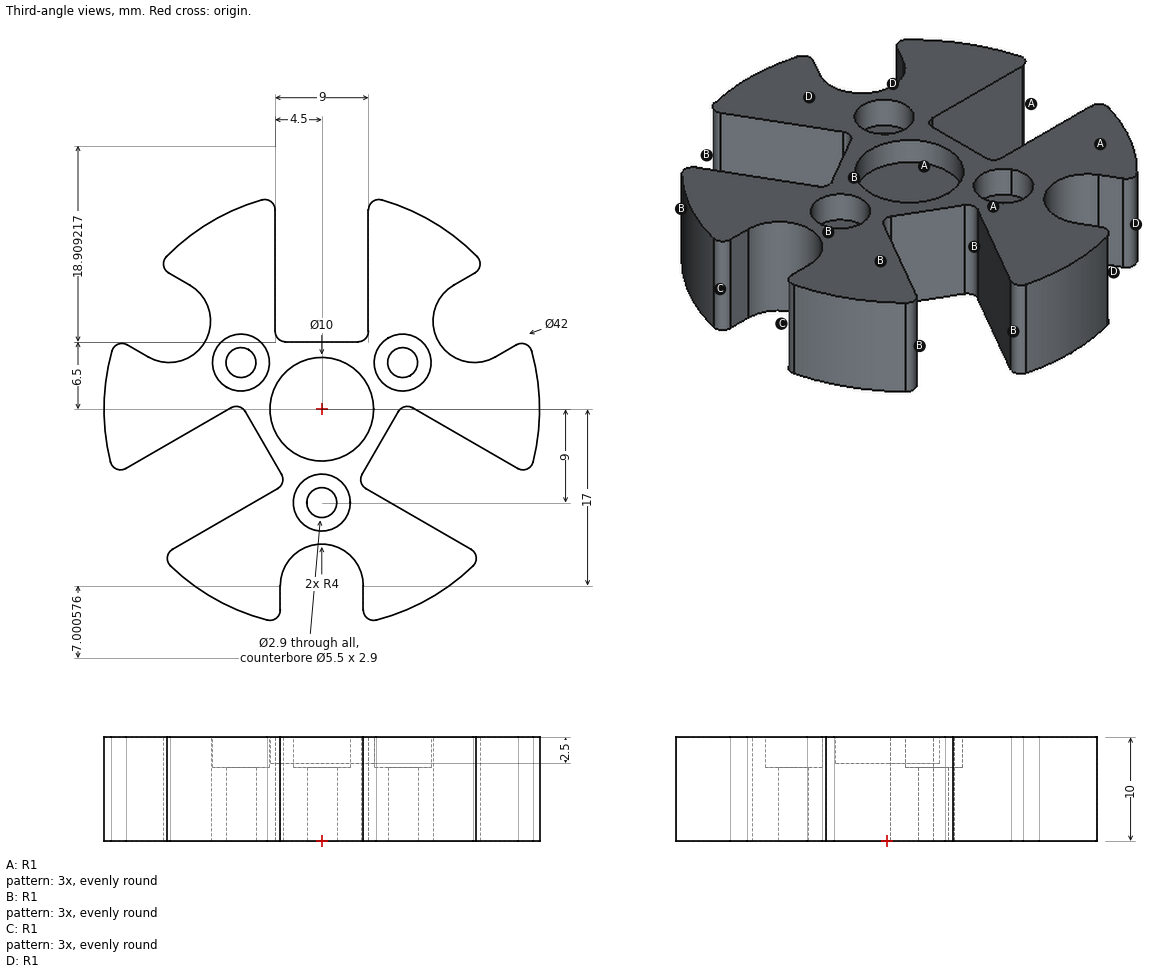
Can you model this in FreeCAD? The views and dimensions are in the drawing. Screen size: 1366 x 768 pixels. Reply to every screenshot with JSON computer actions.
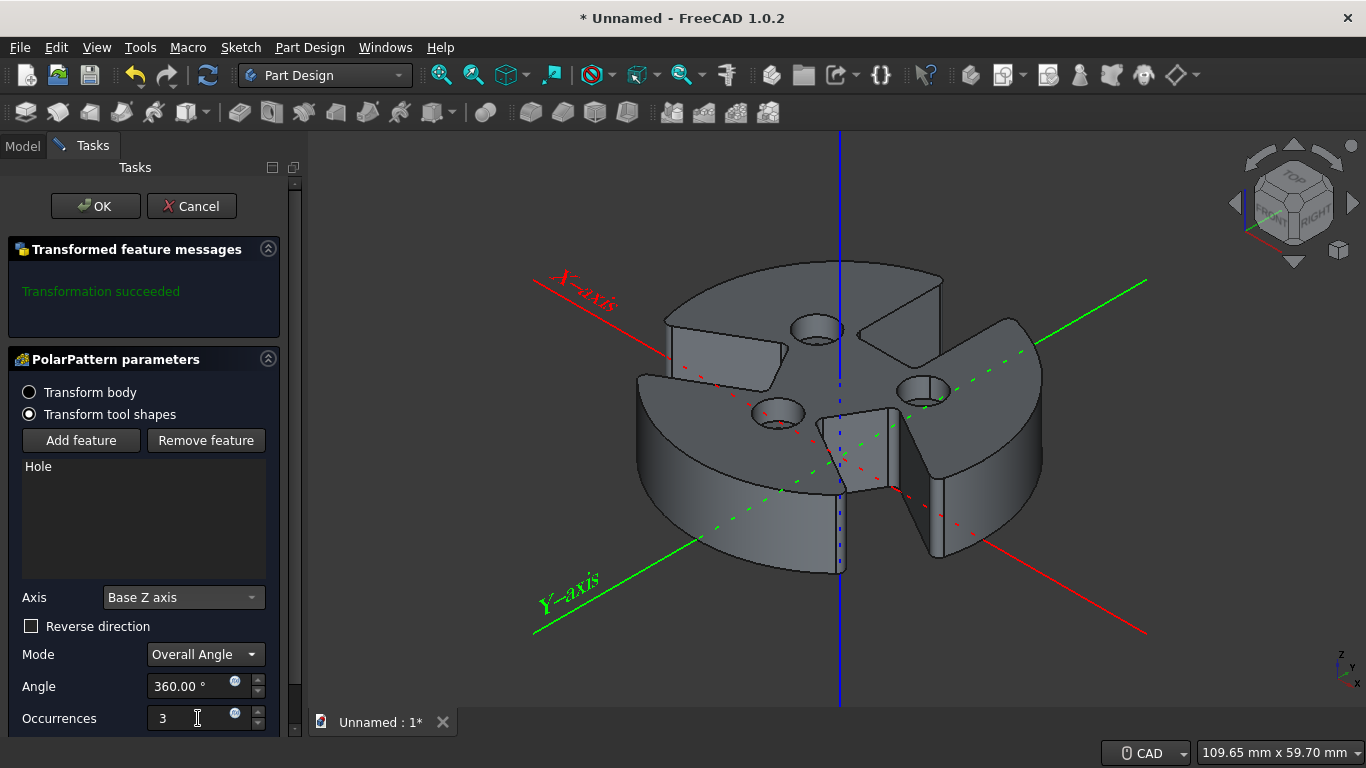
{"action": "left_click", "coordinate": [96, 206]}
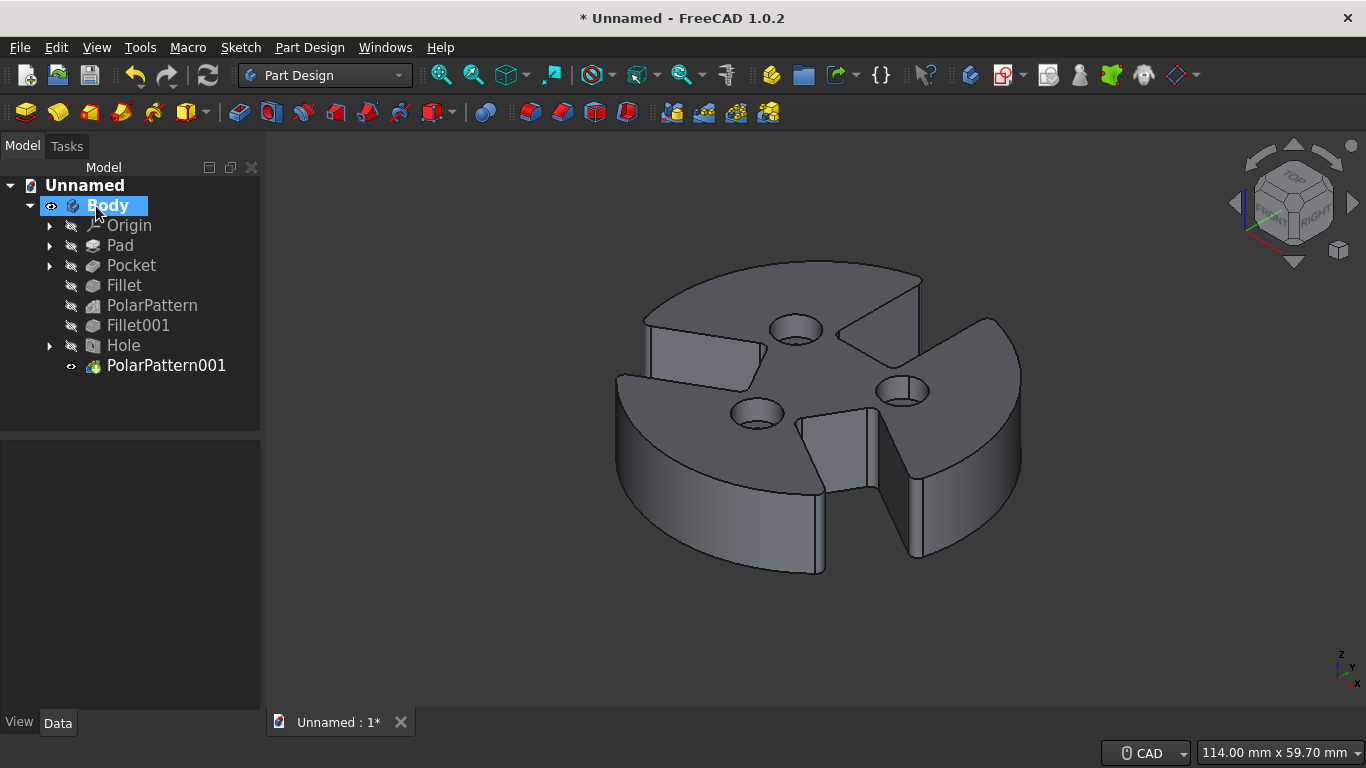
{"action": "left_click", "coordinate": [816, 379]}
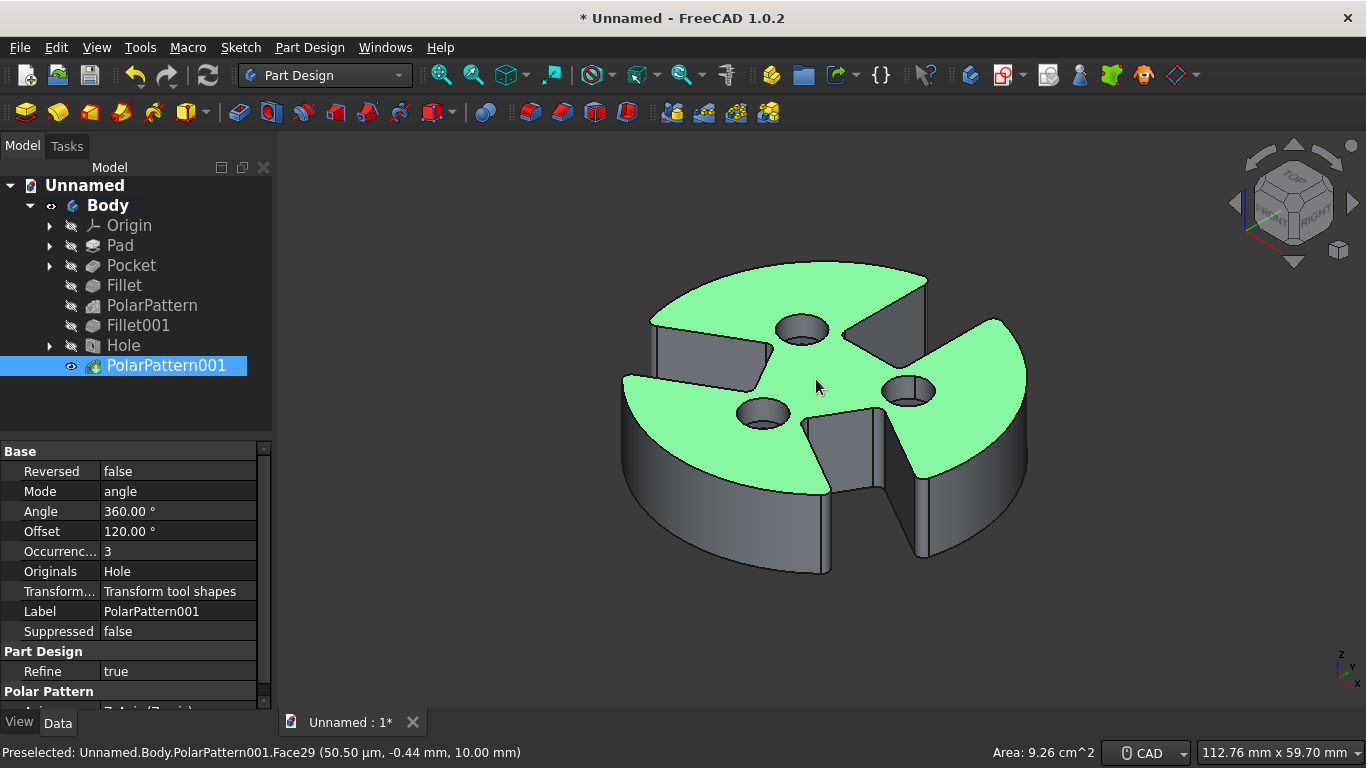
{"action": "left_click", "coordinate": [1004, 76]}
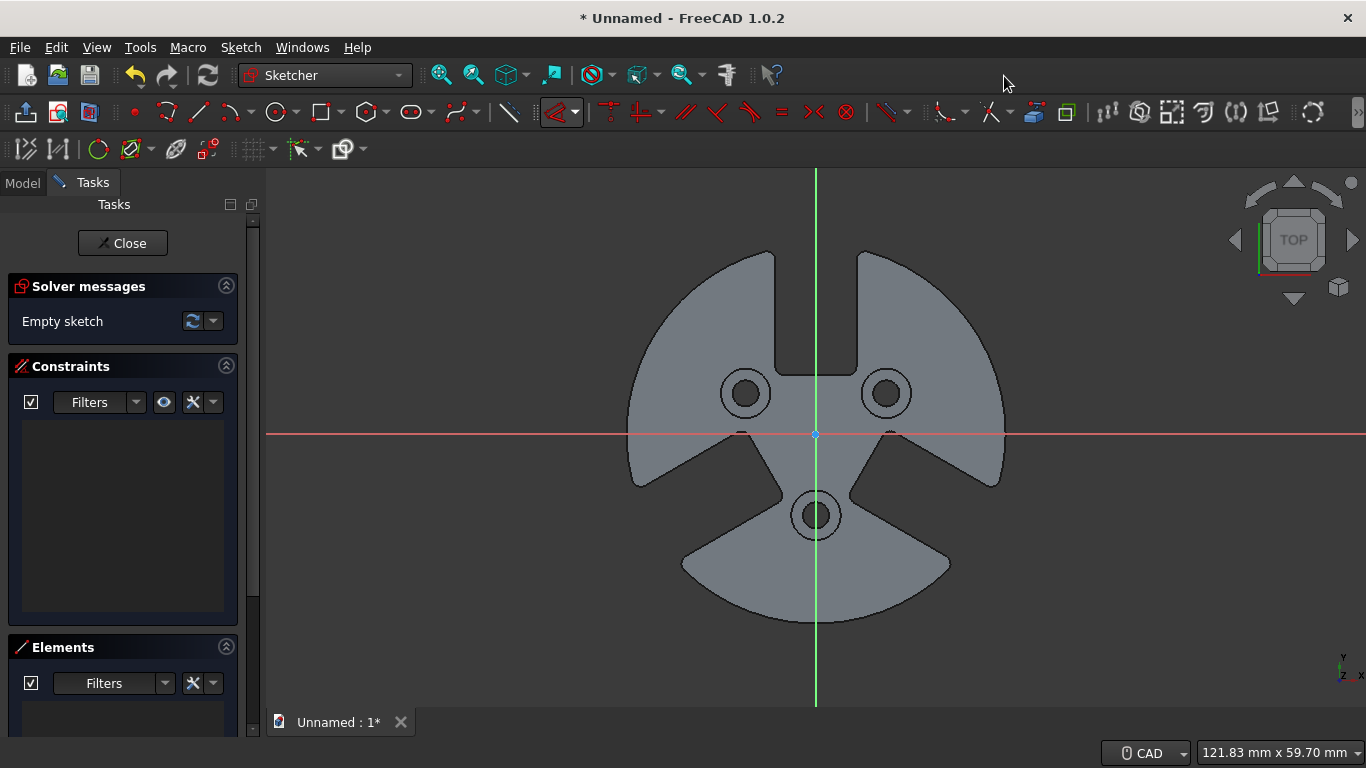
{"action": "scroll", "coordinate": [438, 196], "scroll_direction": "down", "scroll_amount": 1}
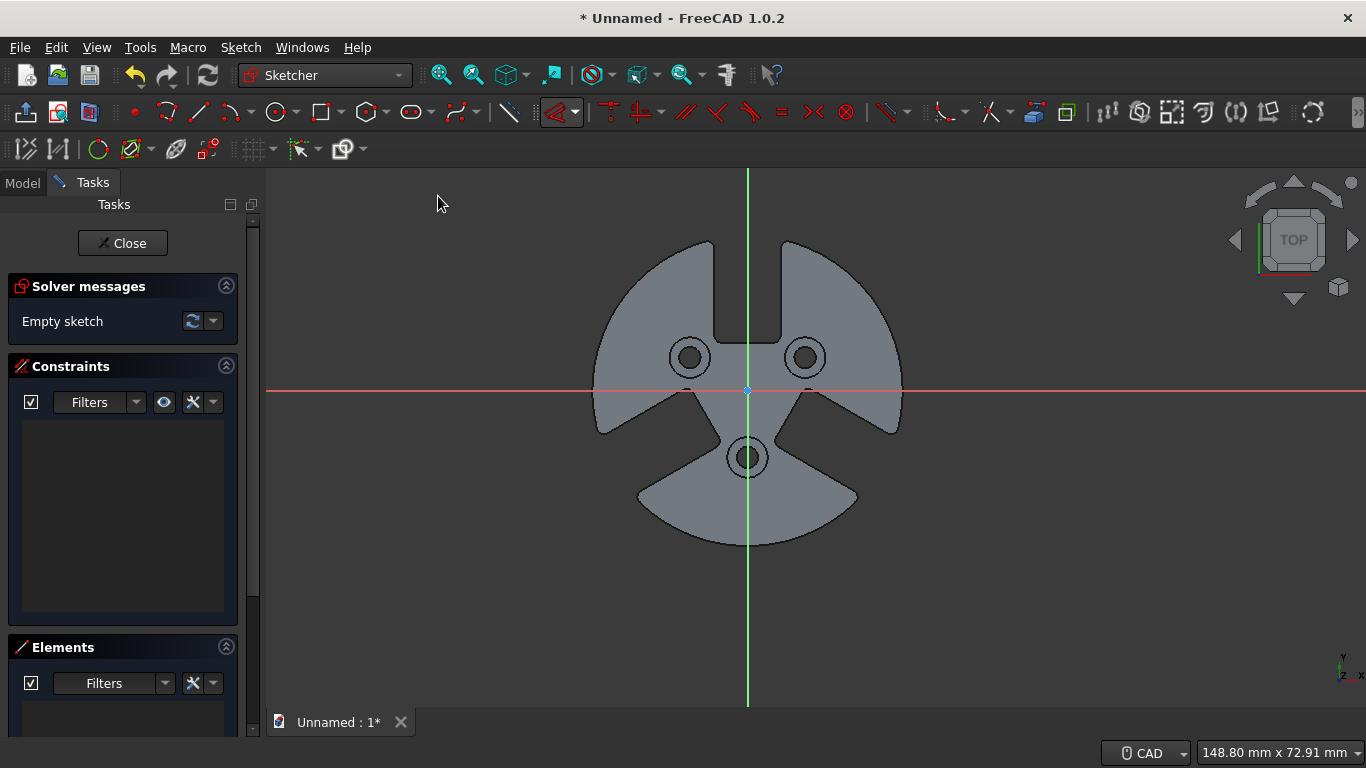
{"action": "scroll", "coordinate": [748, 610], "scroll_direction": "up", "scroll_amount": 2}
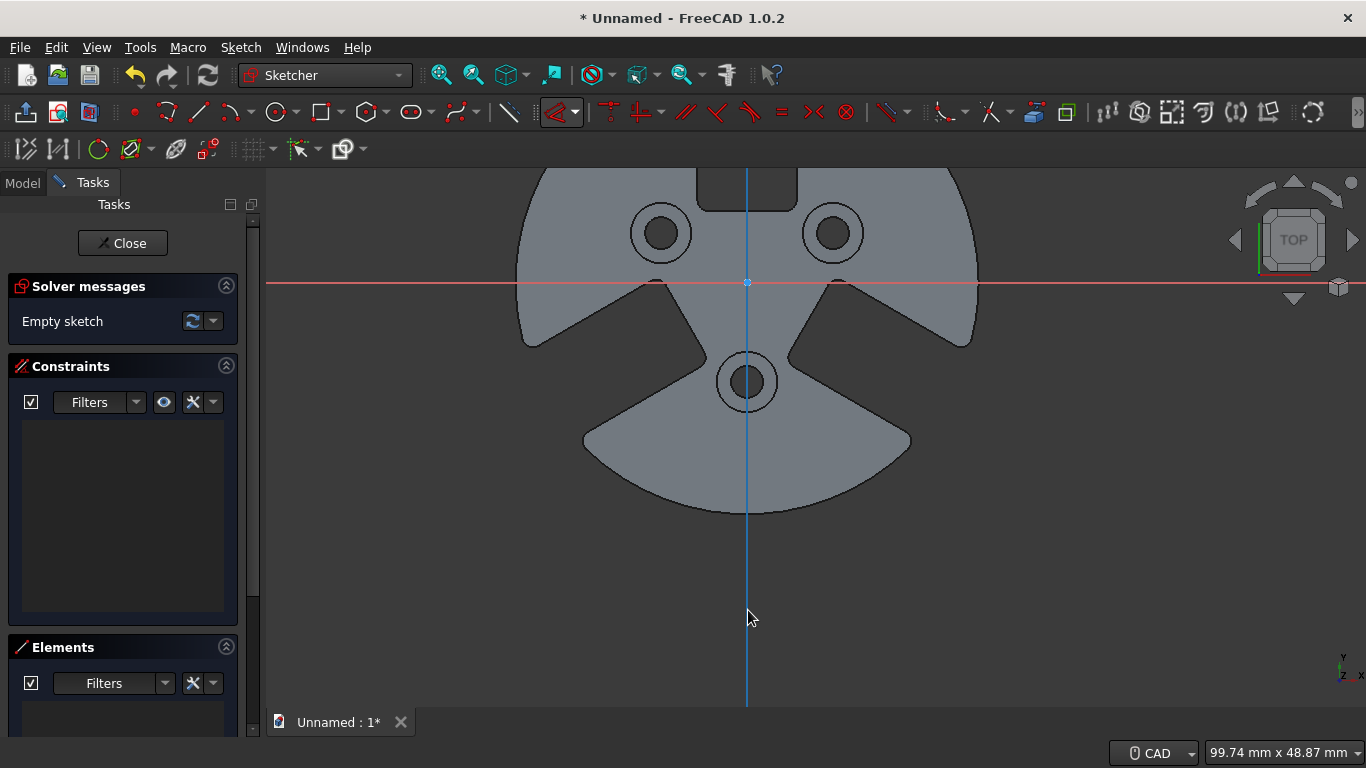
{"action": "left_click", "coordinate": [412, 112]}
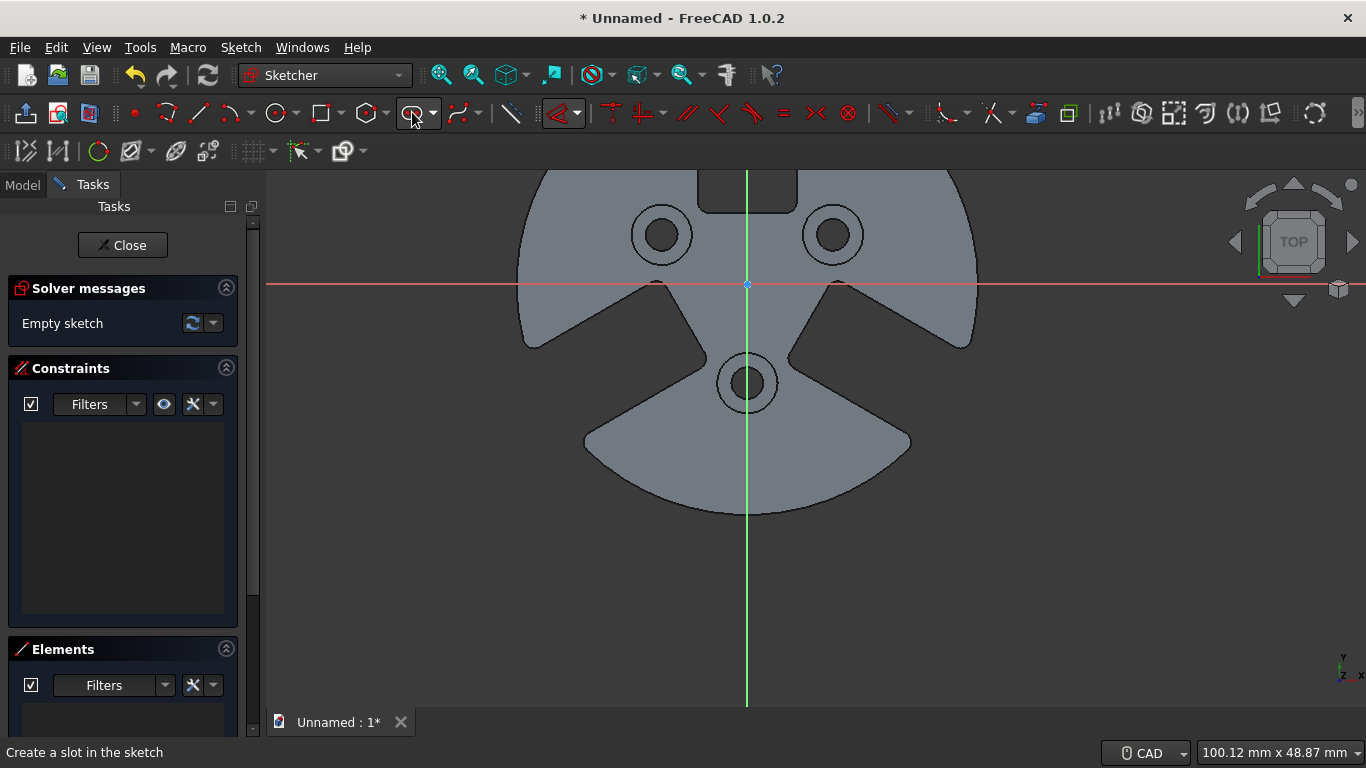
{"action": "left_click", "coordinate": [747, 548]}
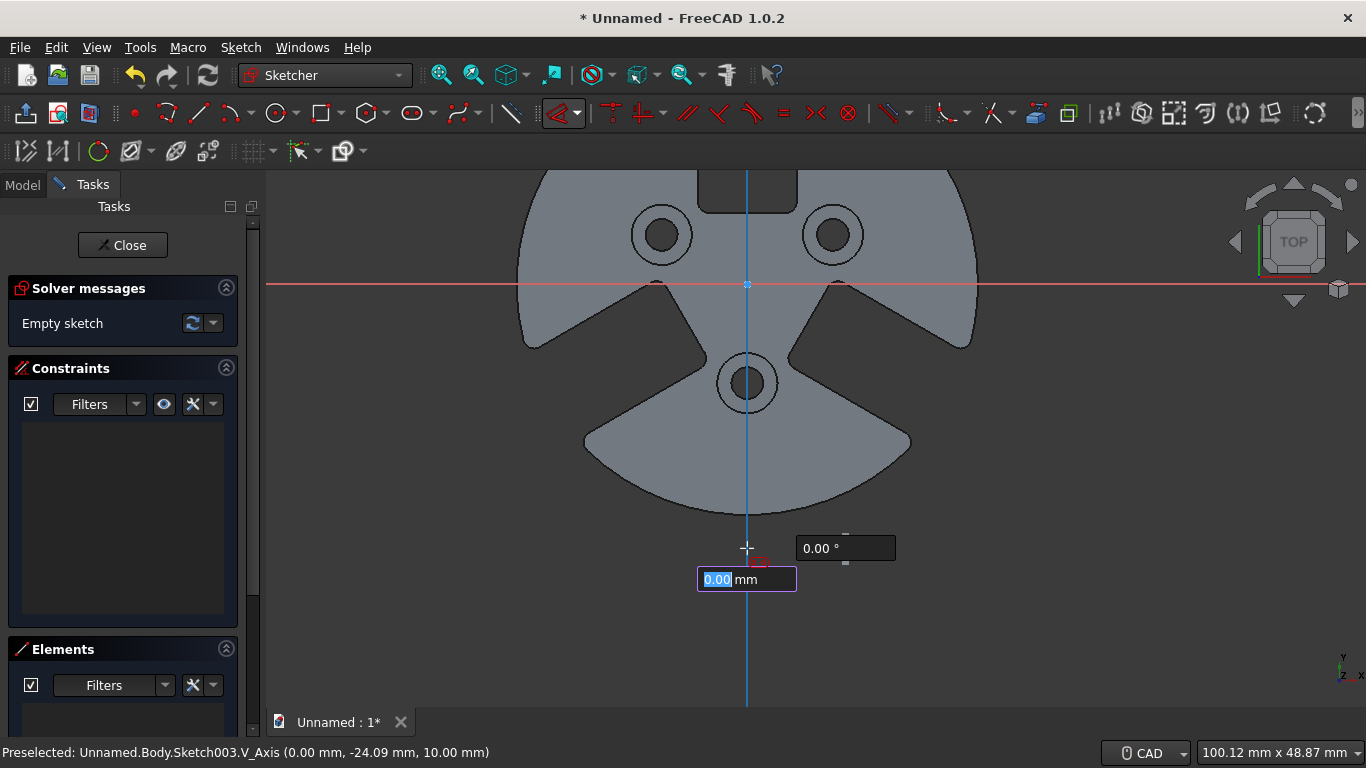
{"action": "left_click", "coordinate": [756, 471]}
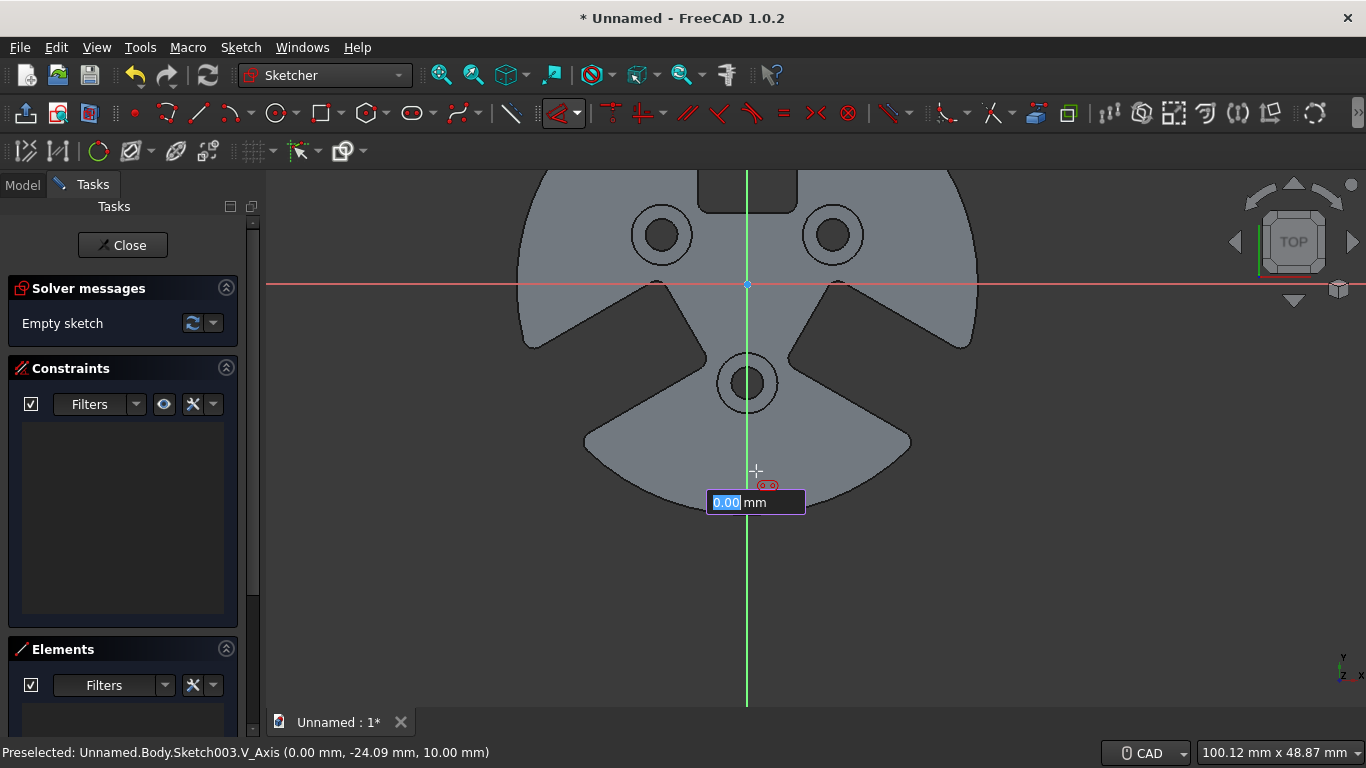
{"action": "left_click", "coordinate": [791, 510]}
{"action": "key", "text": "Escape"}